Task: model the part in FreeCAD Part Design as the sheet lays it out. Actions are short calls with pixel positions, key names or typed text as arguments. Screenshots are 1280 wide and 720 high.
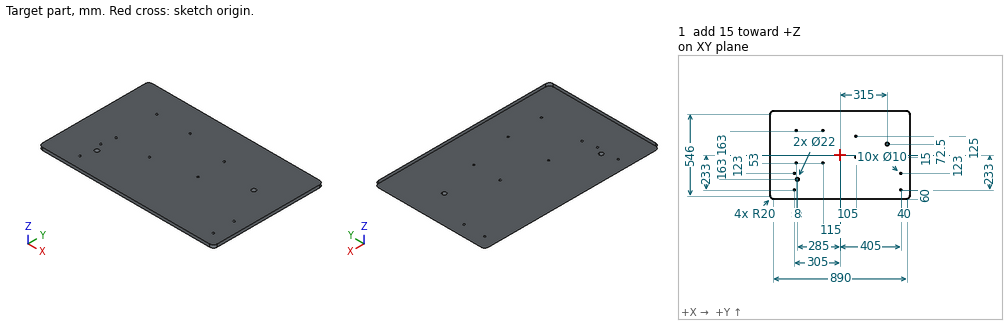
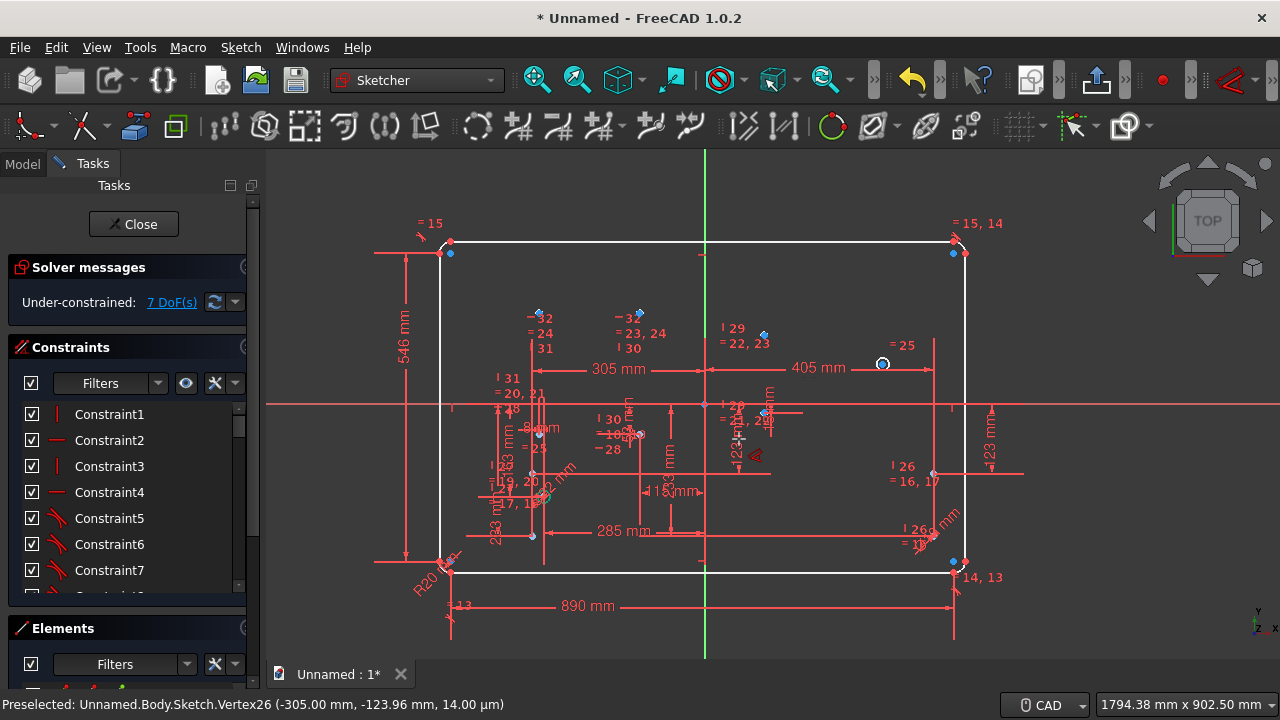
click(764, 413)
click(734, 370)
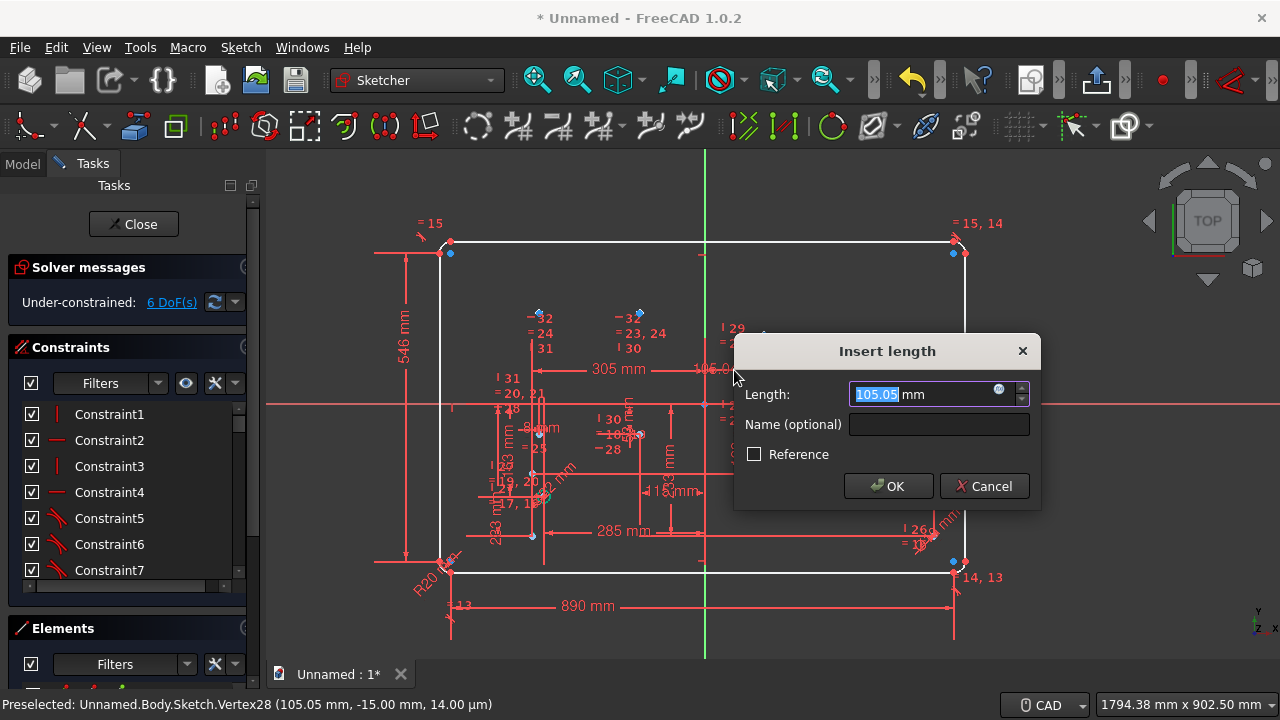
text(105)
key(Return)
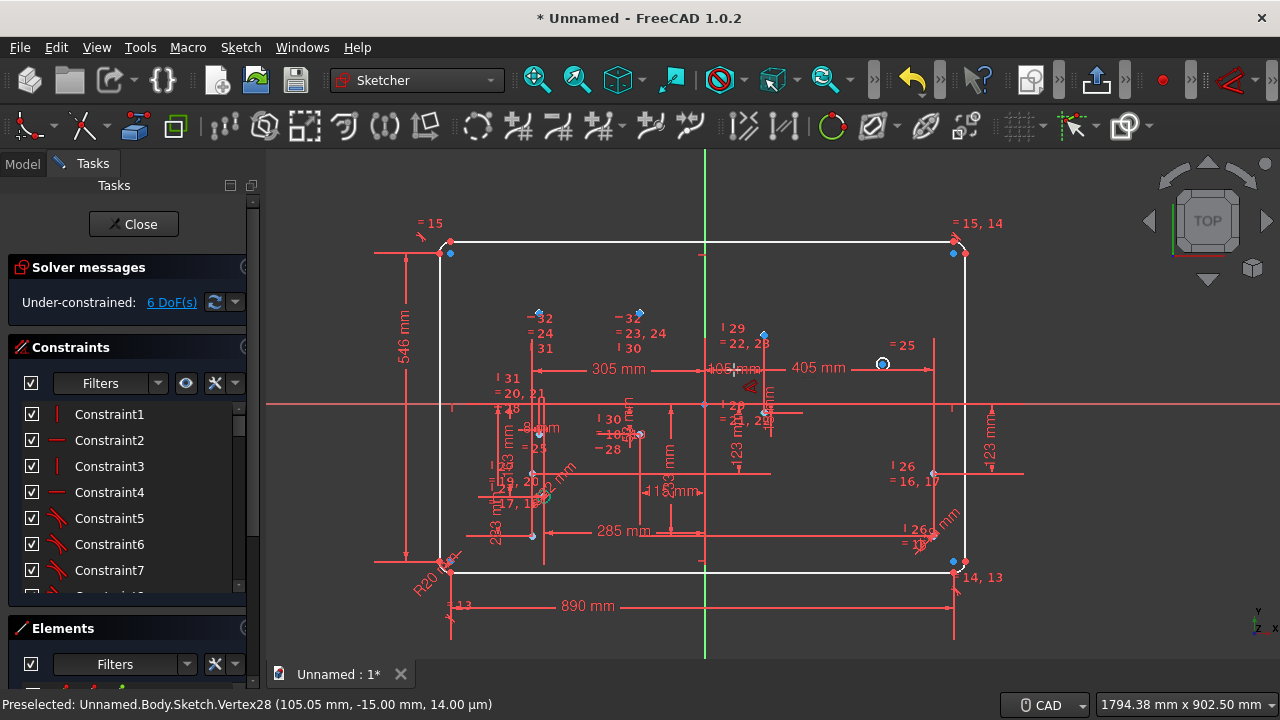
click(883, 364)
click(794, 330)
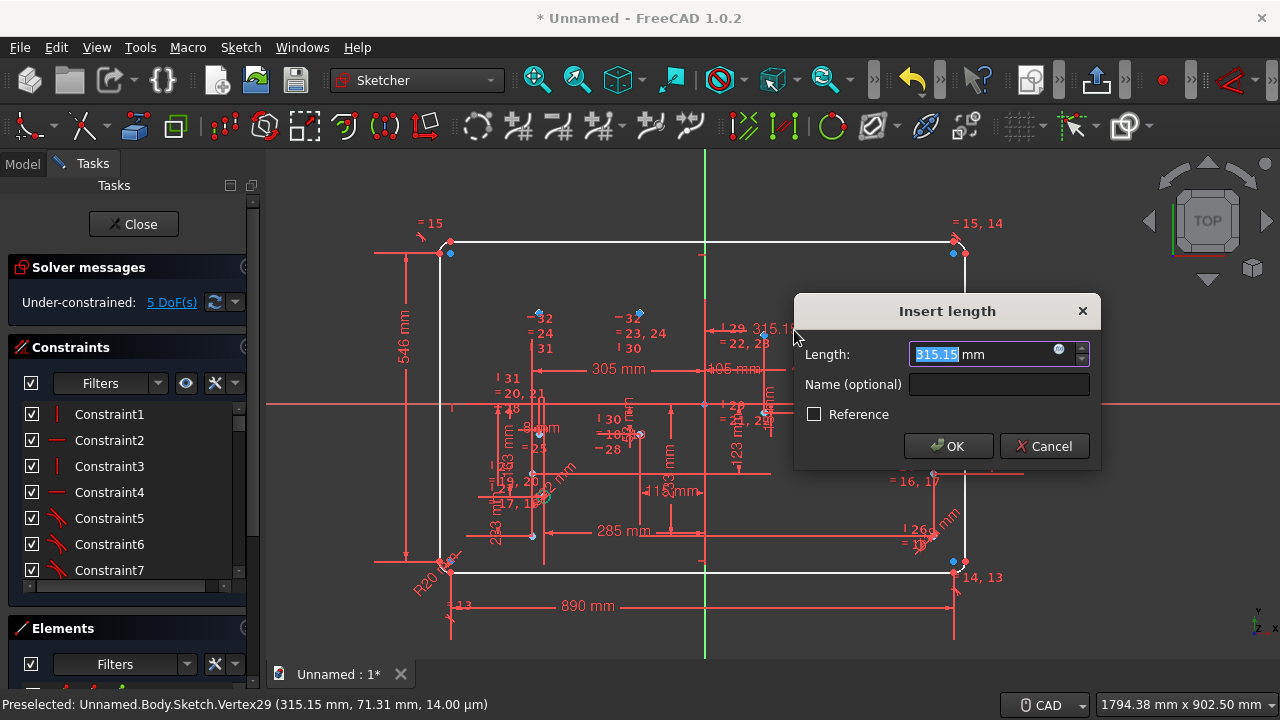
text(315)
key(Return)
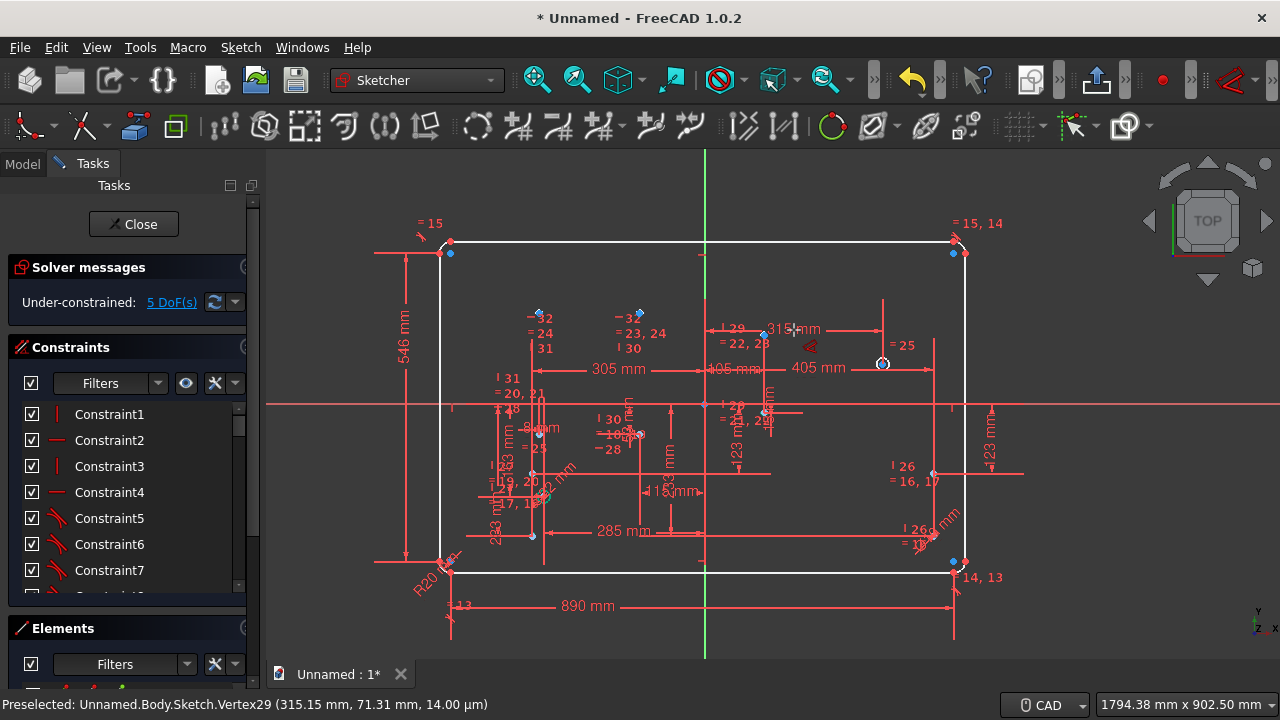
click(764, 335)
click(671, 345)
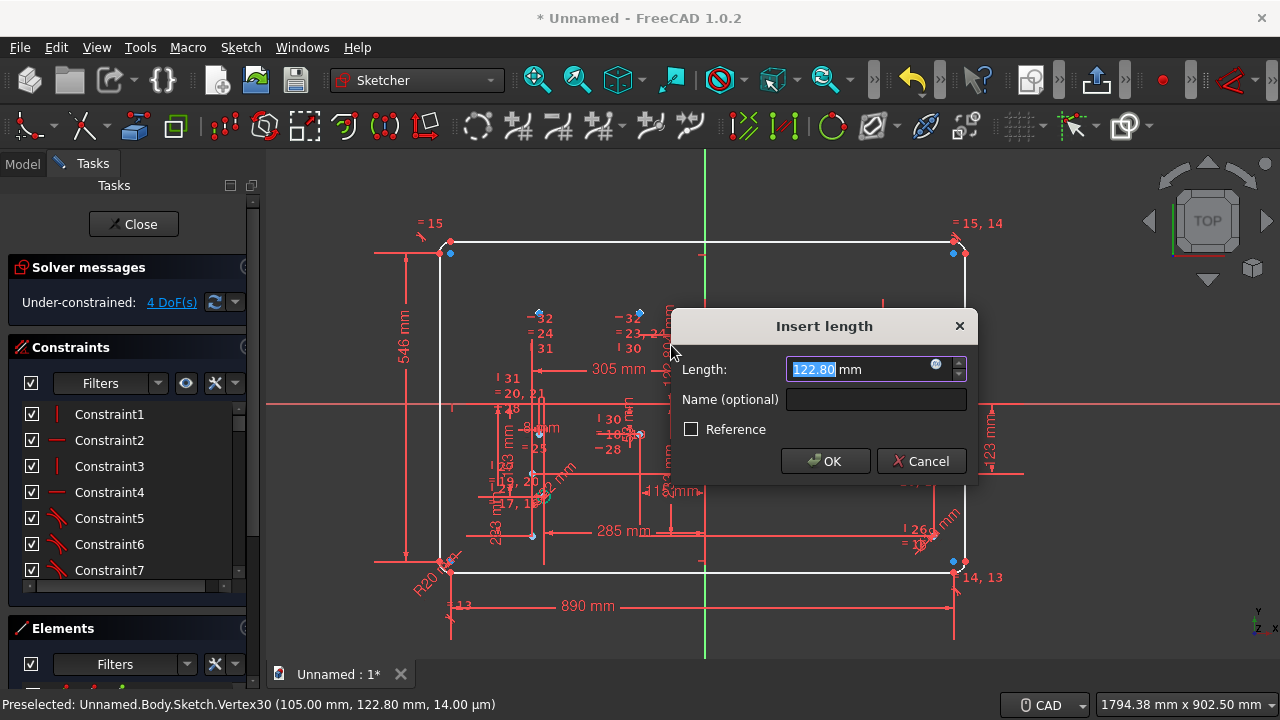
text(125)
key(Return)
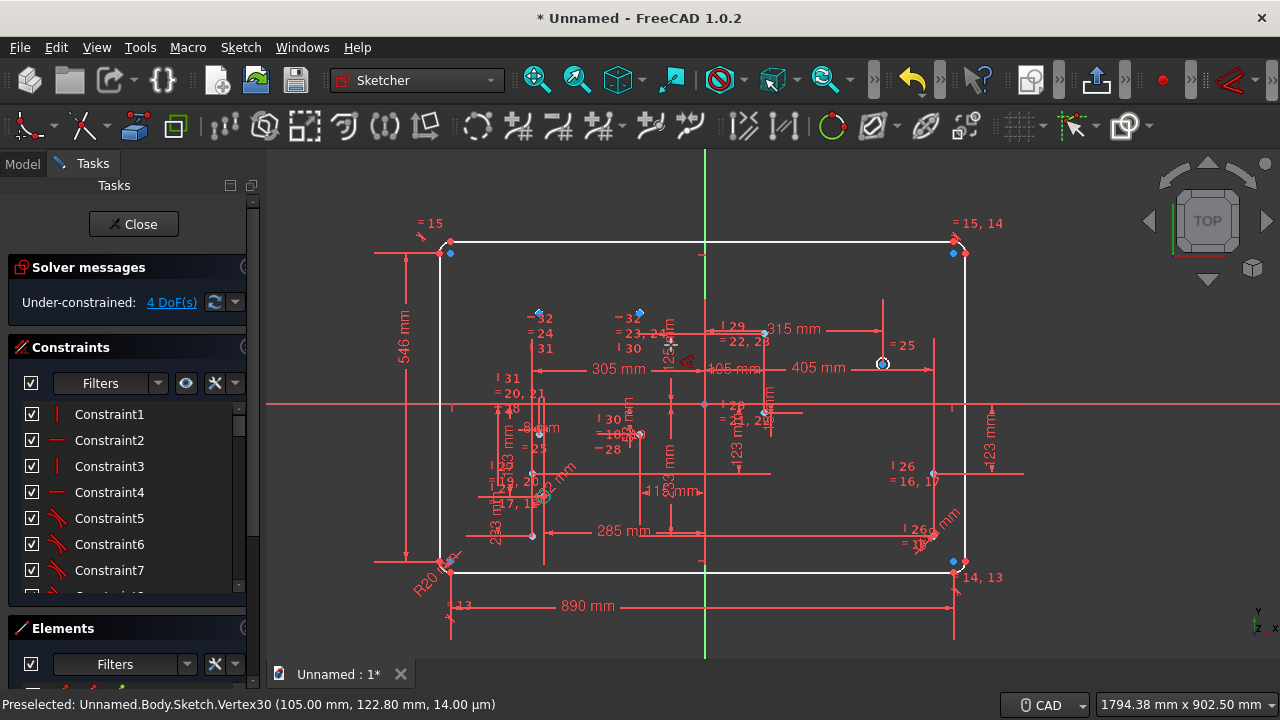
click(640, 313)
click(606, 391)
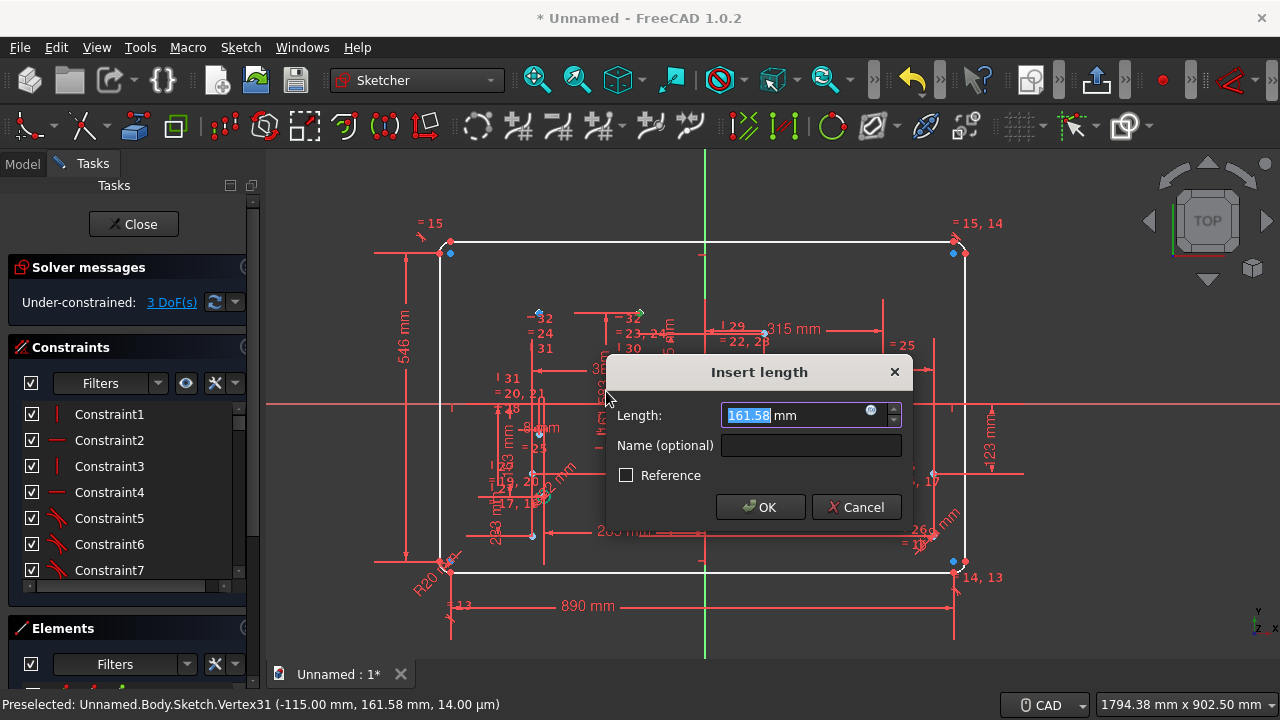
text(163)
key(Return)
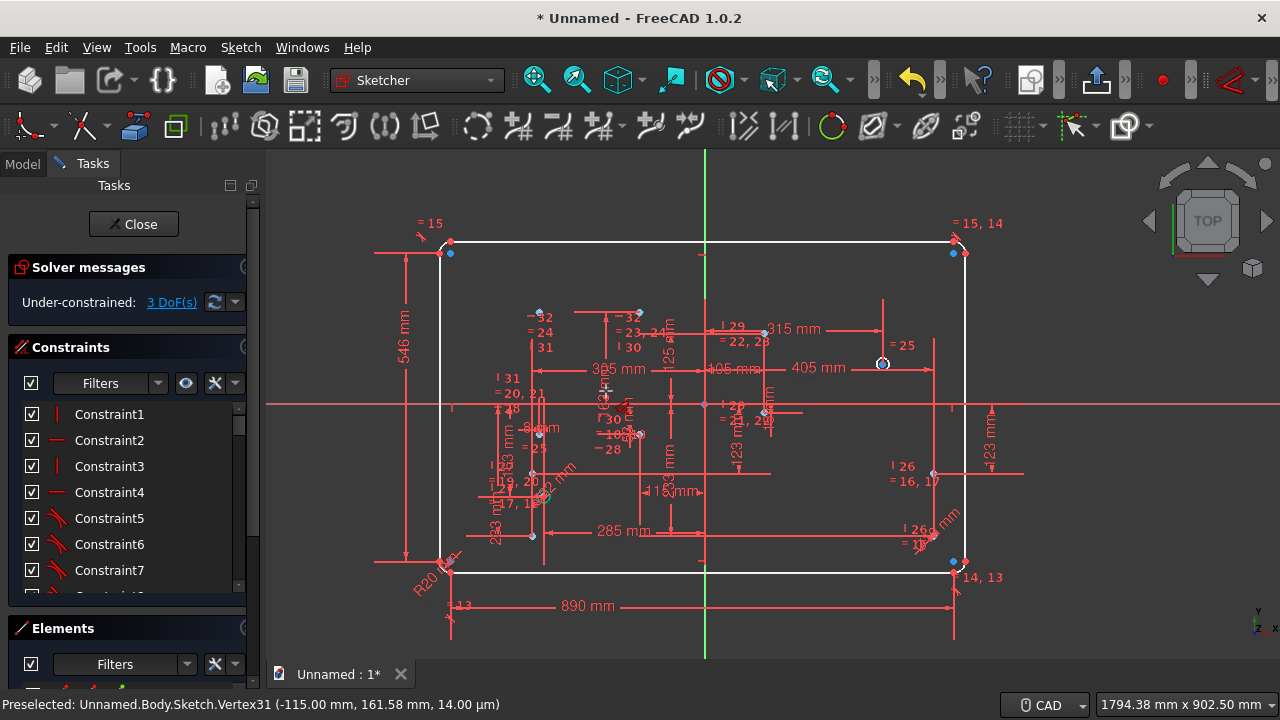
scroll(954, 573, up, 3)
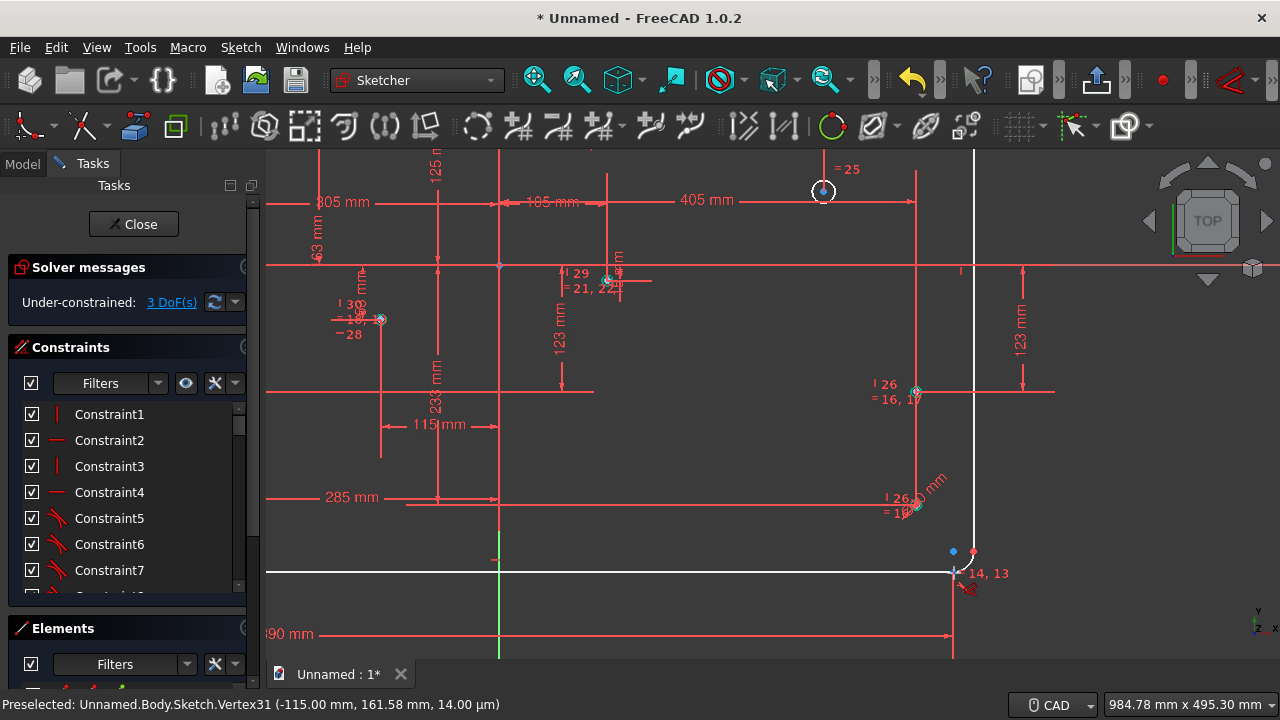
click(953, 572)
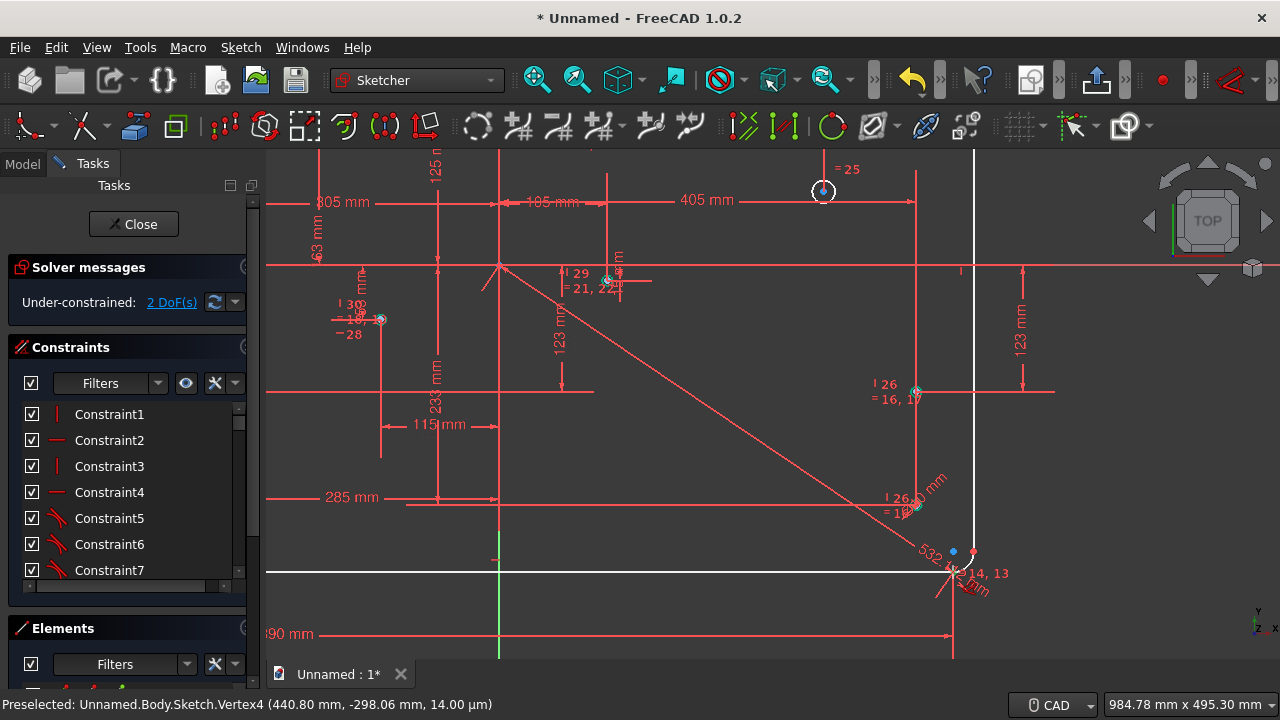
click(916, 505)
click(935, 606)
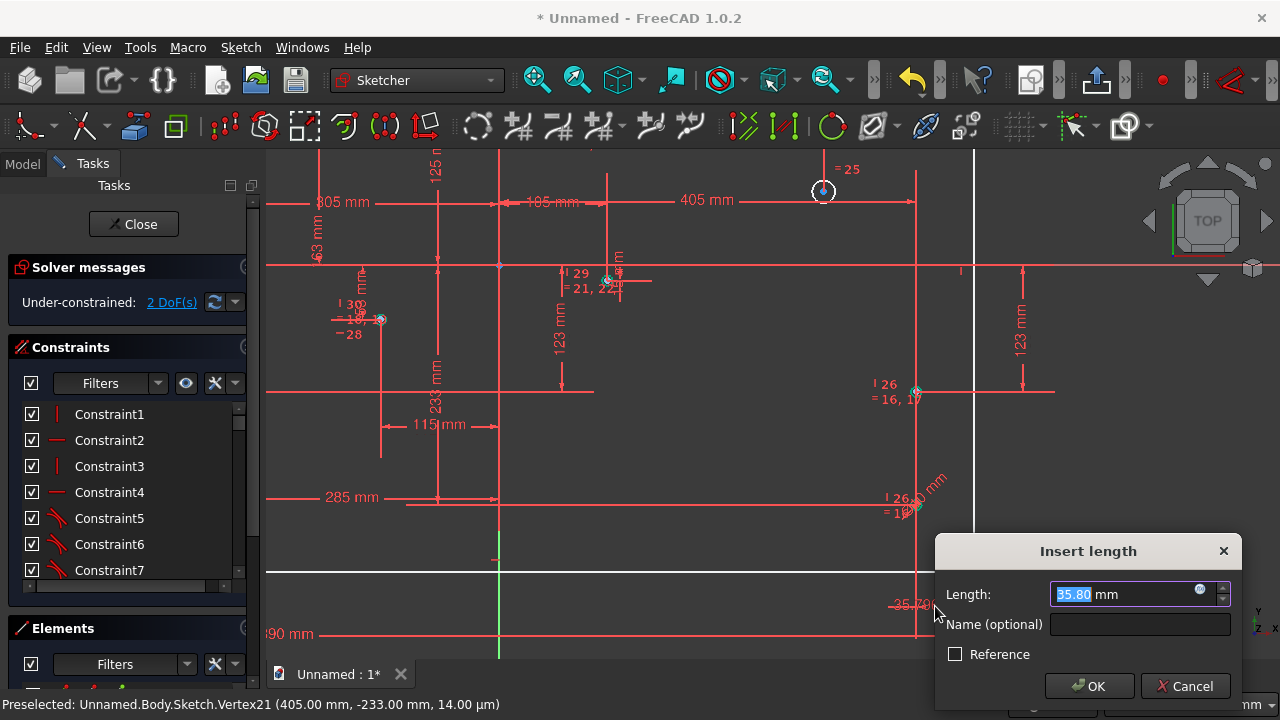
text(40)
key(Return)